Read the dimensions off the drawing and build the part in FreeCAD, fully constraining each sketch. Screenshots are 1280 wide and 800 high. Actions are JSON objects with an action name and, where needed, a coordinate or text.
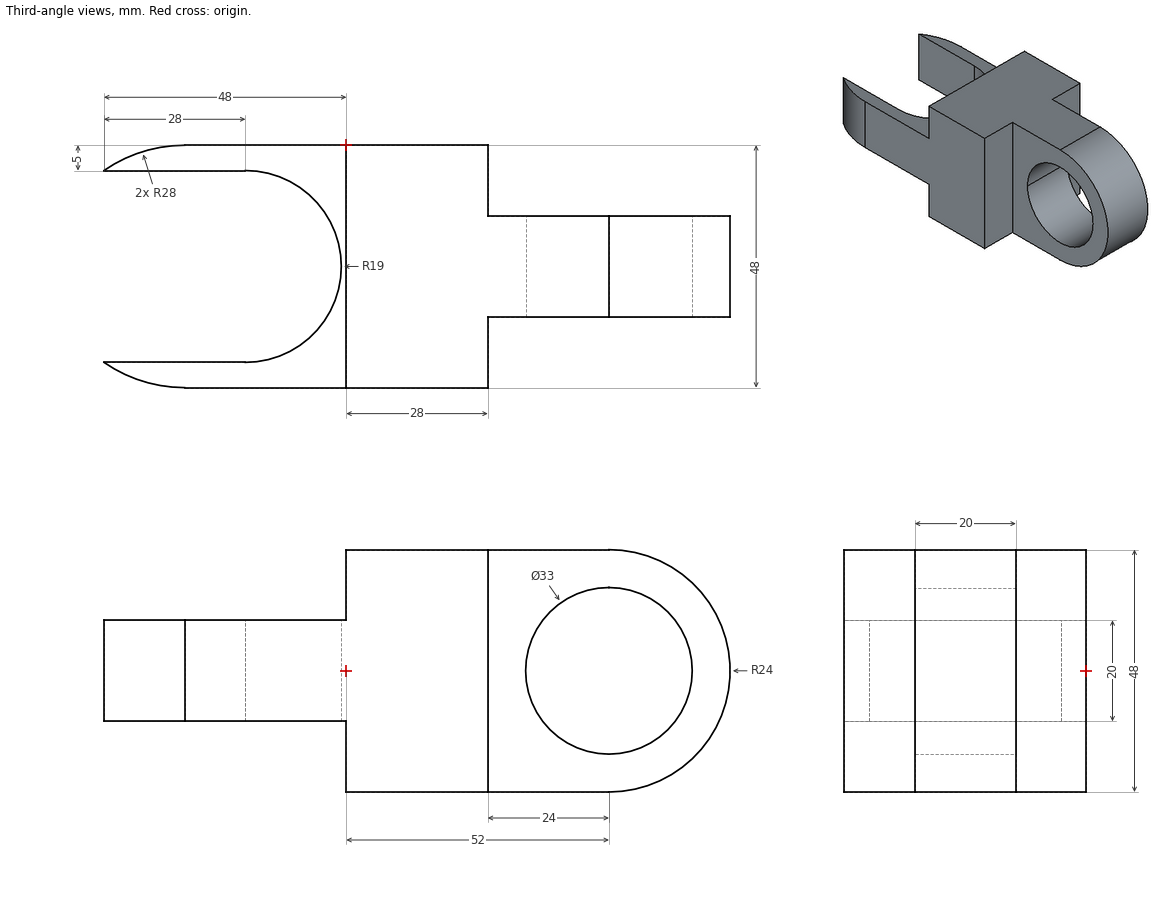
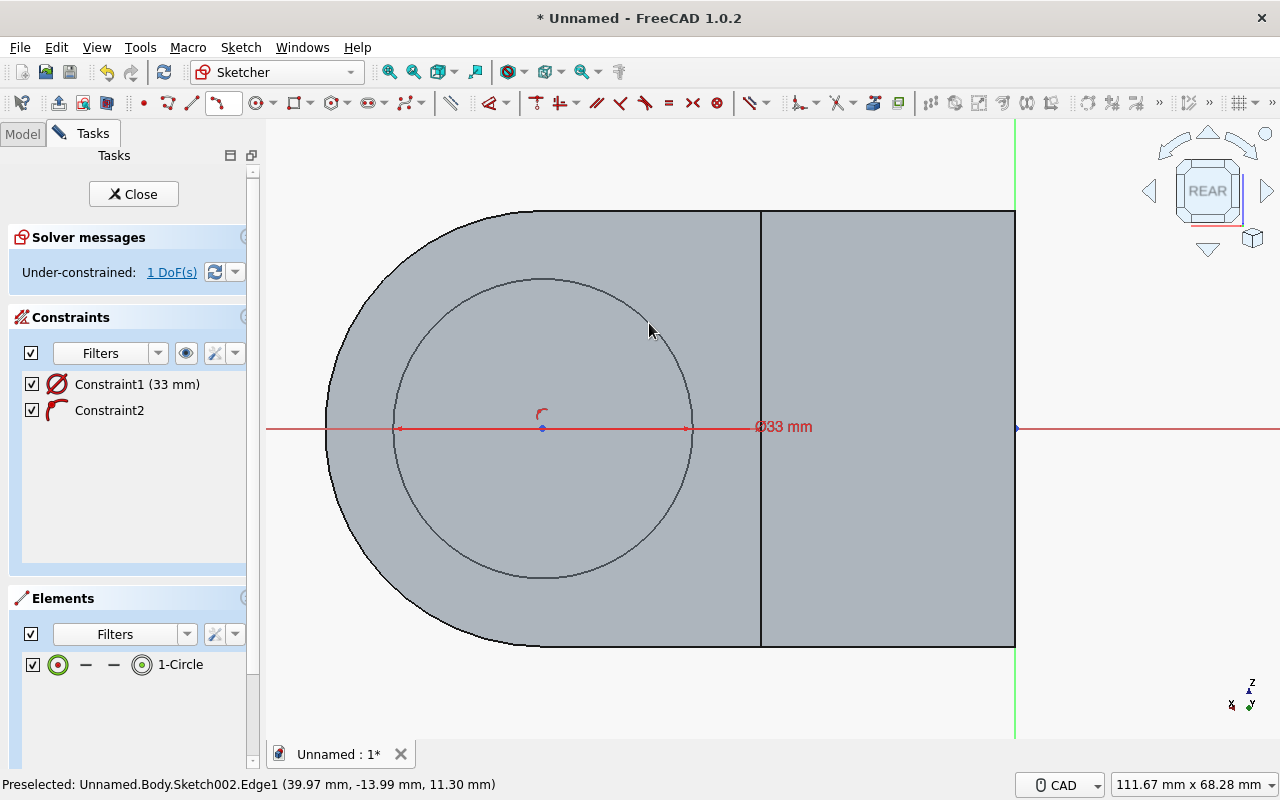
{"action": "left_click", "coordinate": [490, 104]}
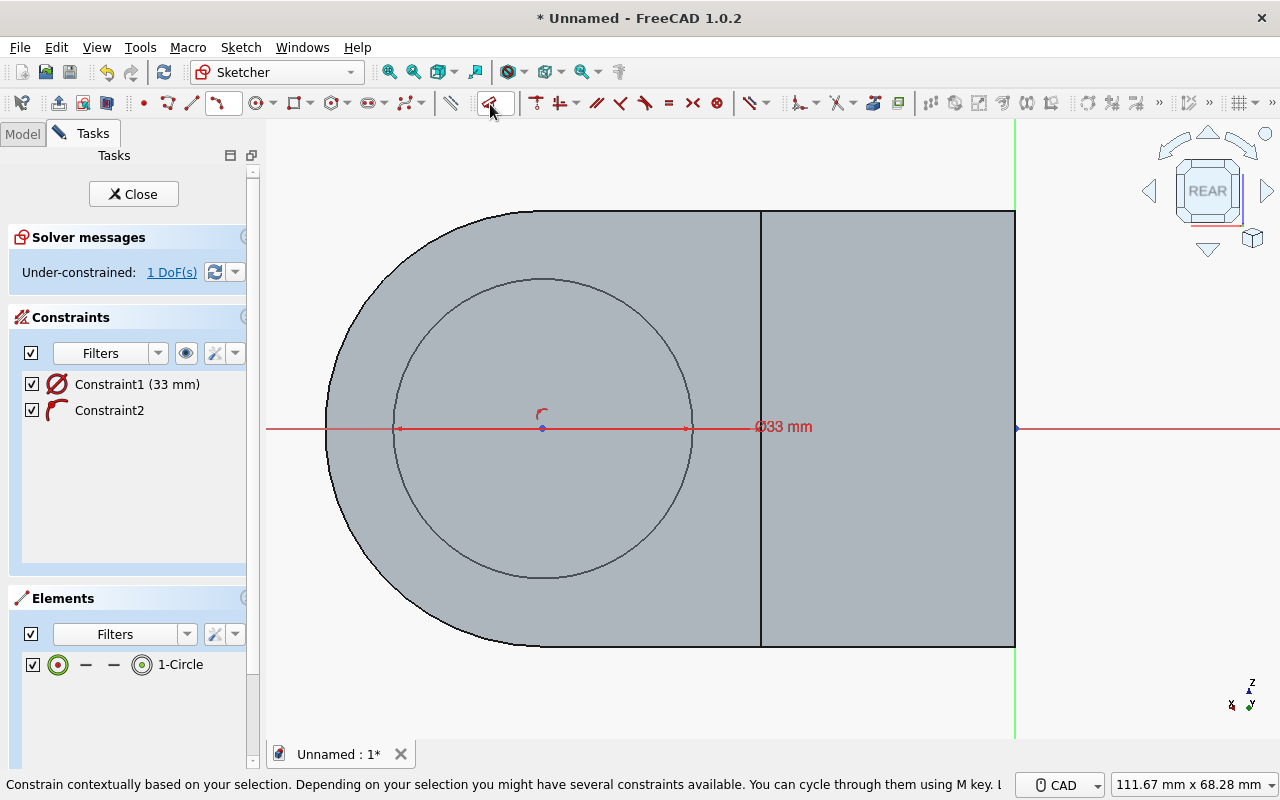
{"action": "left_click", "coordinate": [543, 429]}
{"action": "left_click", "coordinate": [779, 463]}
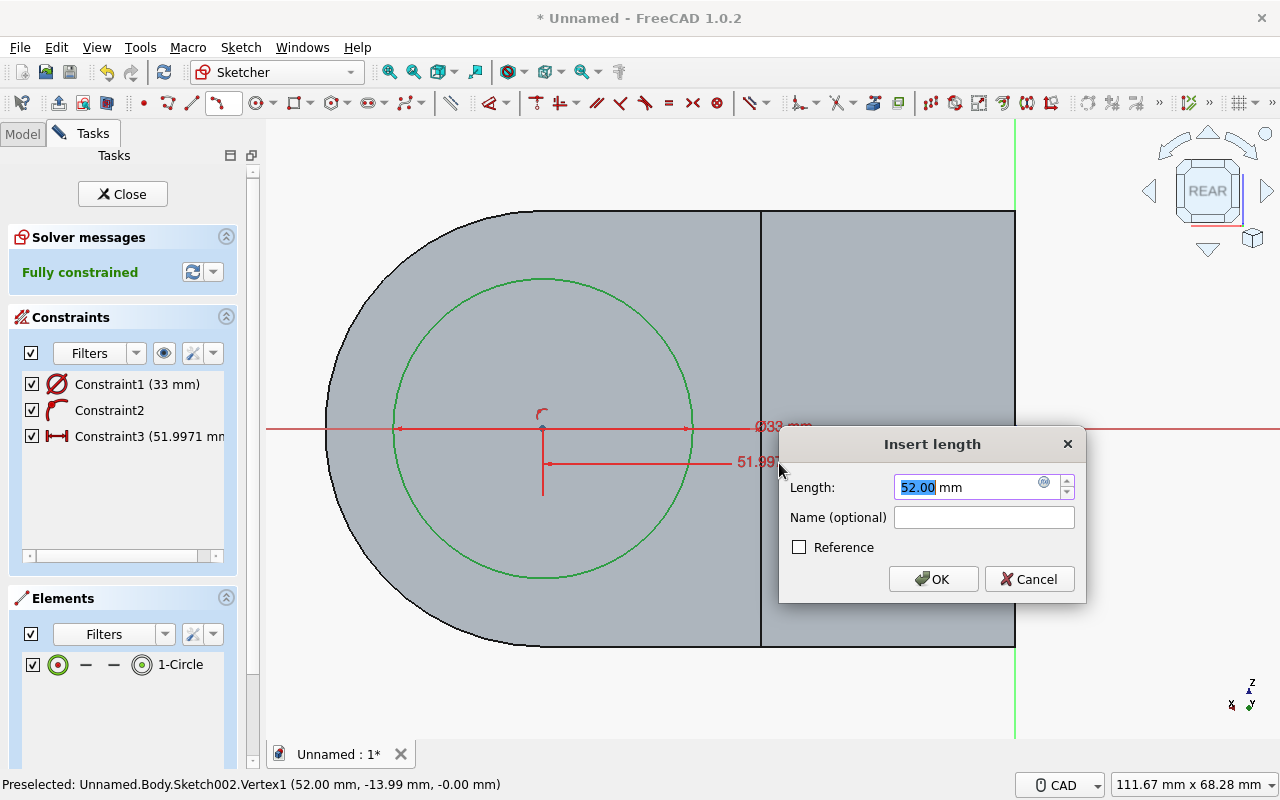
{"action": "type", "text": "52"}
{"action": "key", "text": "Return"}
{"action": "key", "text": "Escape"}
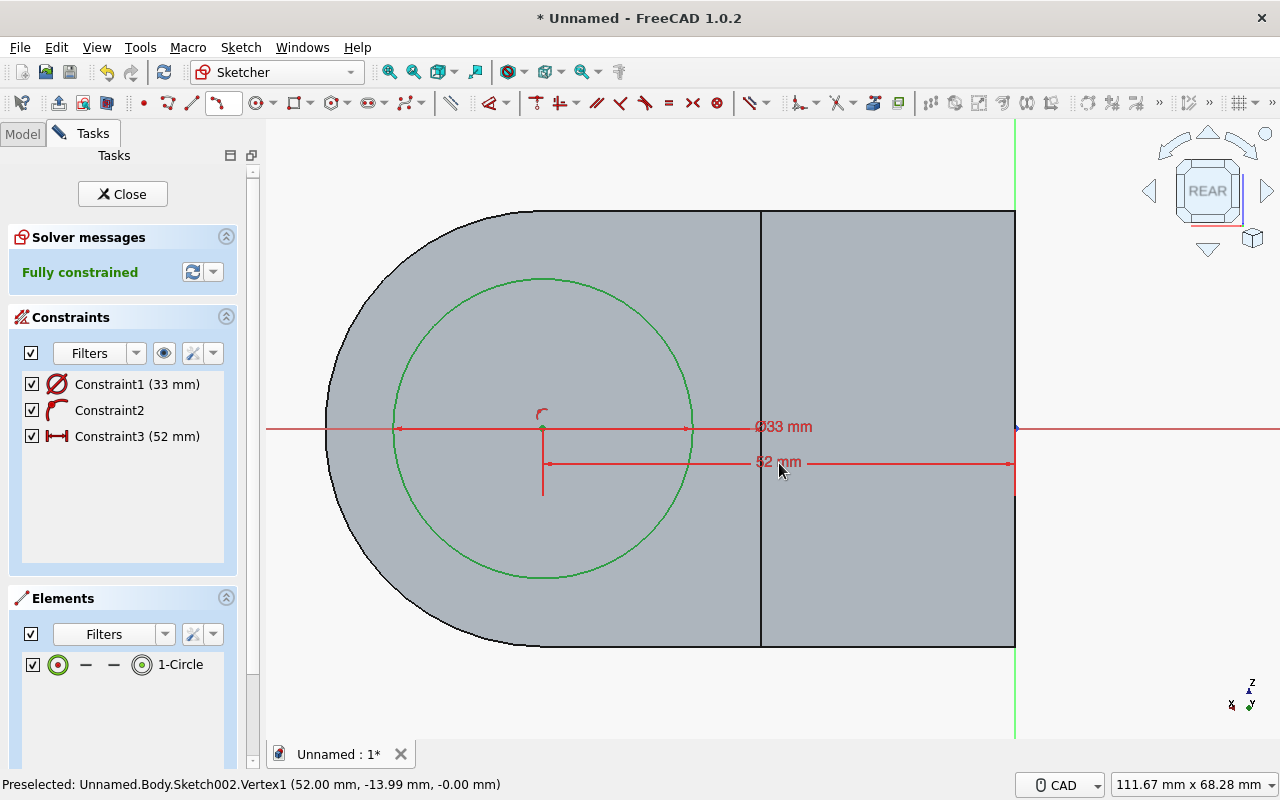
{"action": "left_click", "coordinate": [123, 194]}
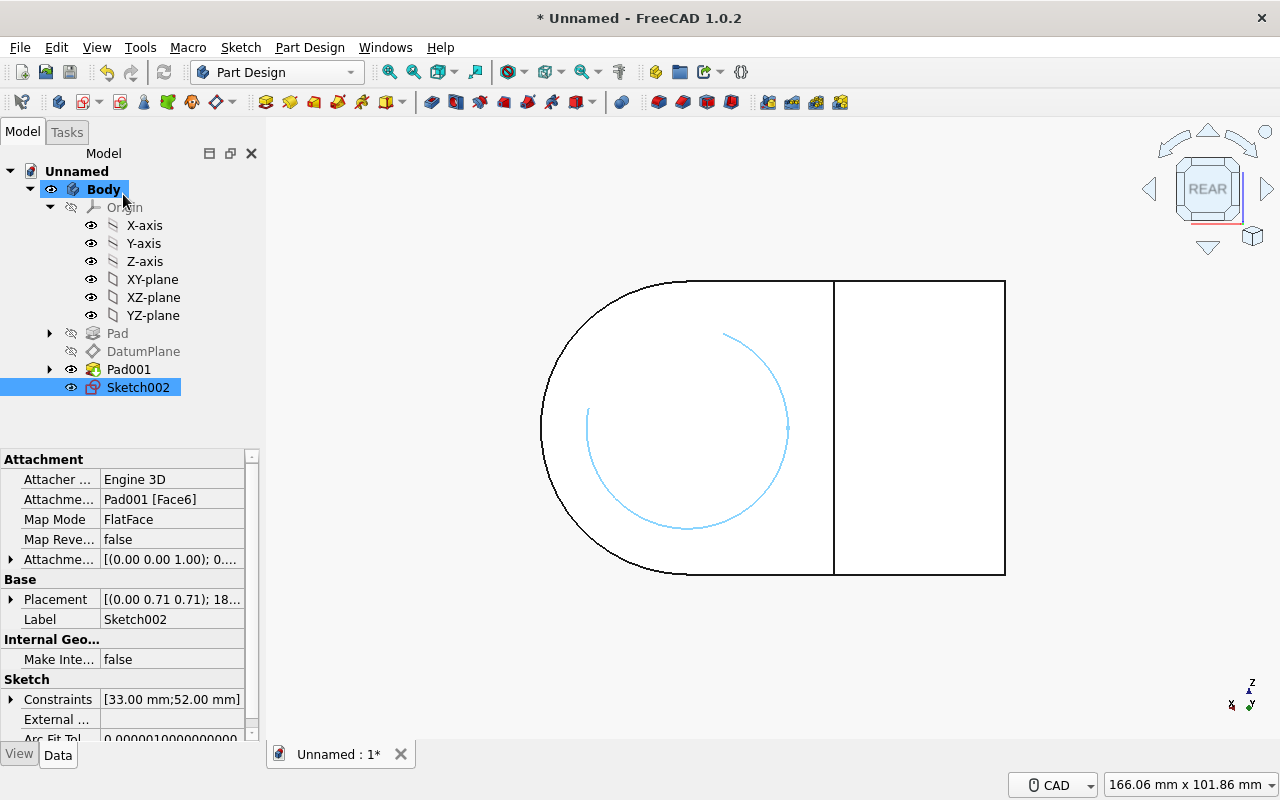
{"action": "left_click", "coordinate": [432, 102]}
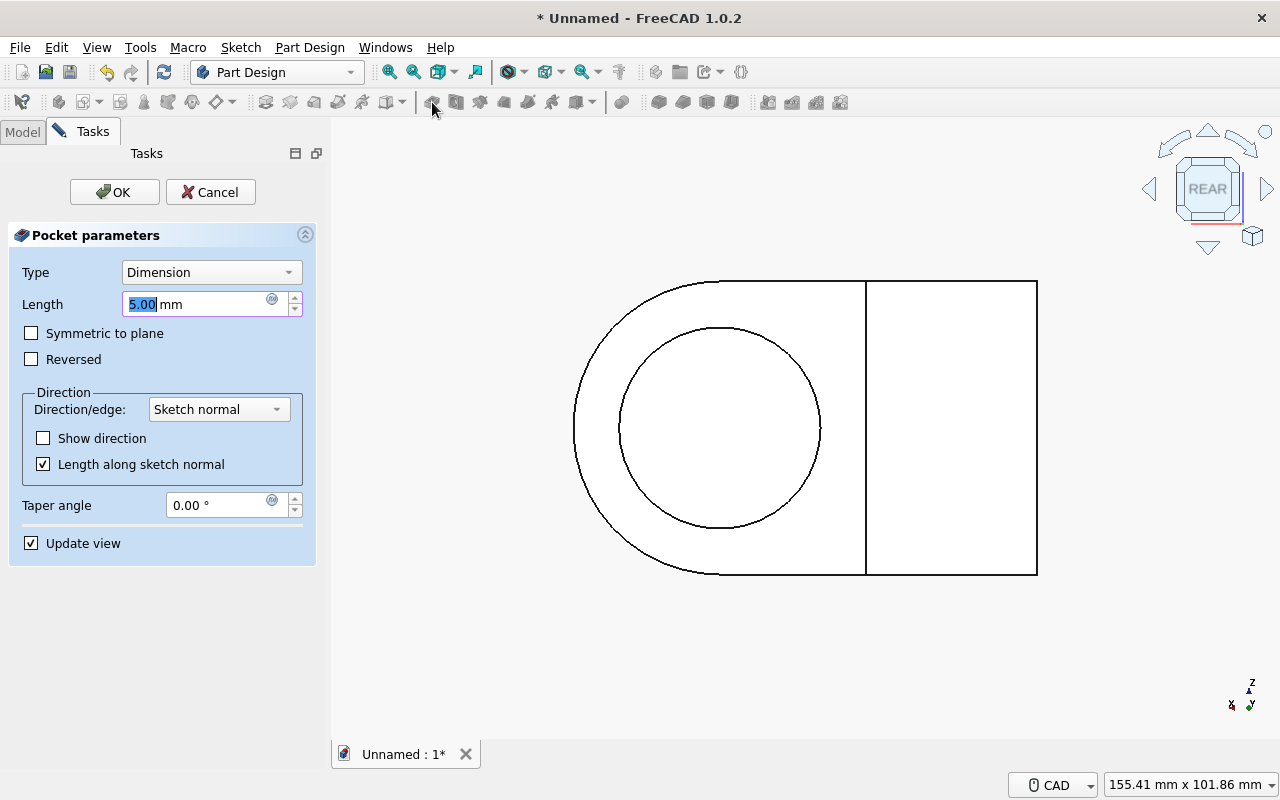
{"action": "type", "text": "20"}
{"action": "key", "text": "Tab"}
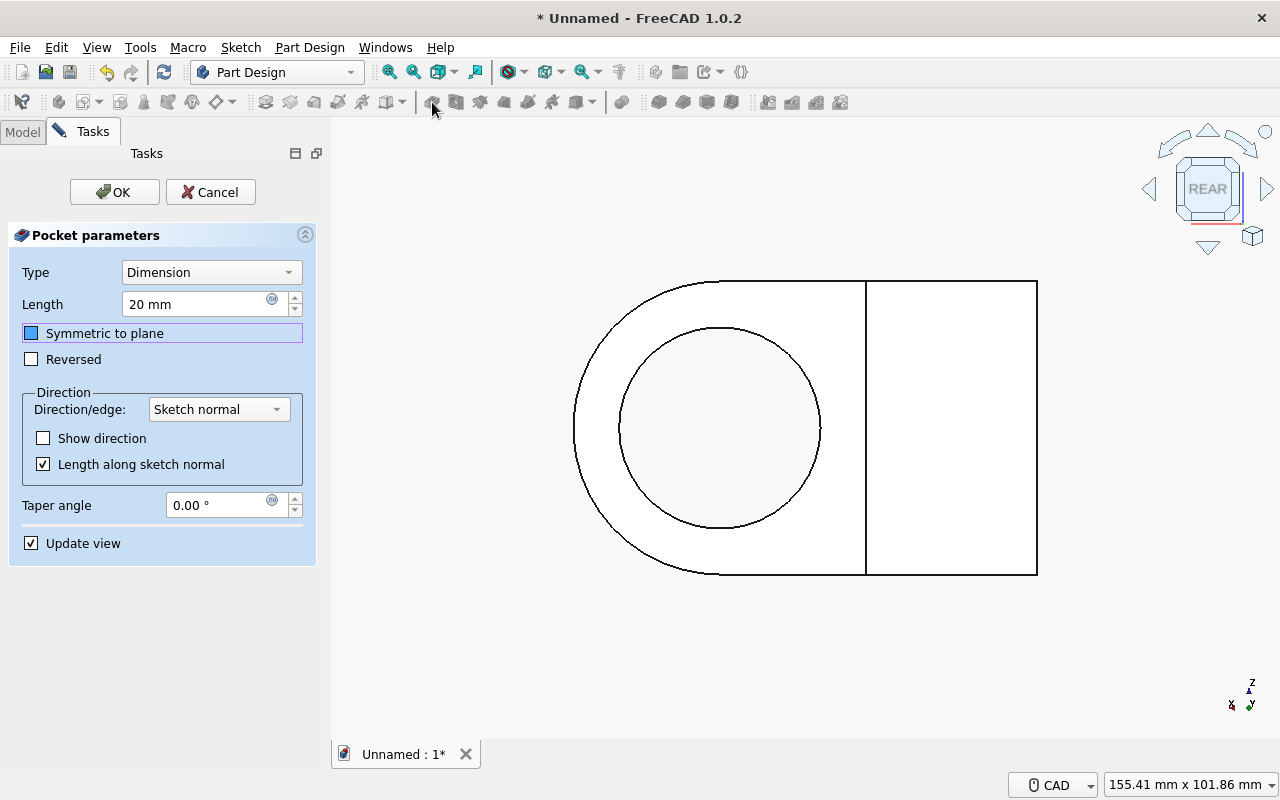
{"action": "left_click", "coordinate": [115, 192]}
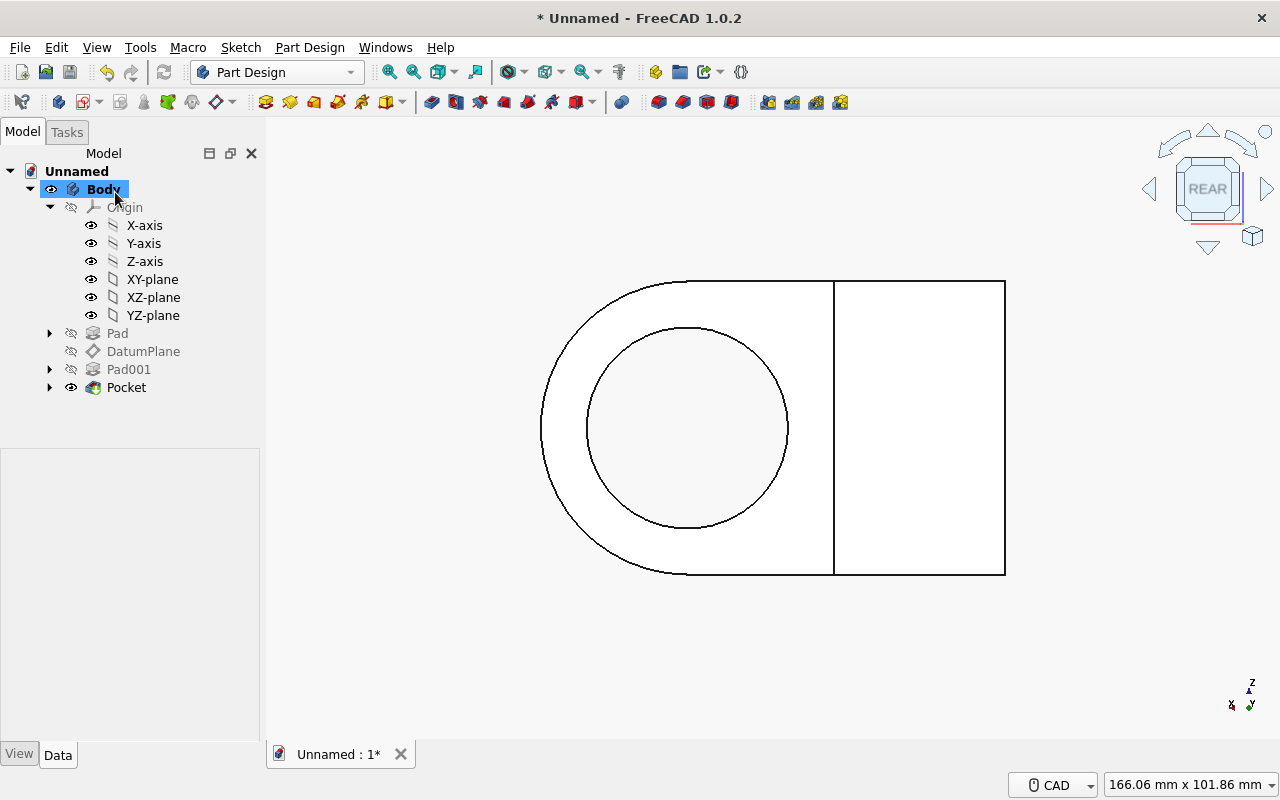
{"action": "left_click", "coordinate": [84, 102]}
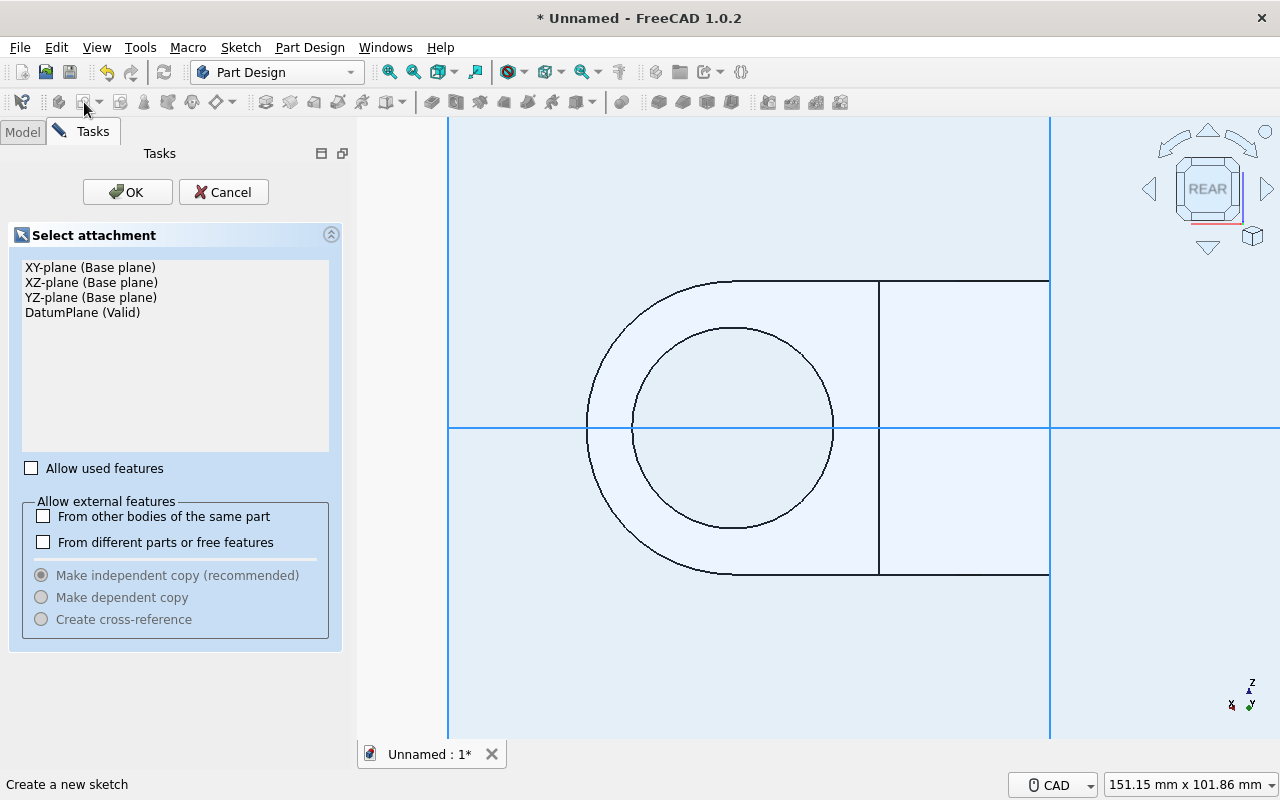
{"action": "left_click", "coordinate": [82, 268]}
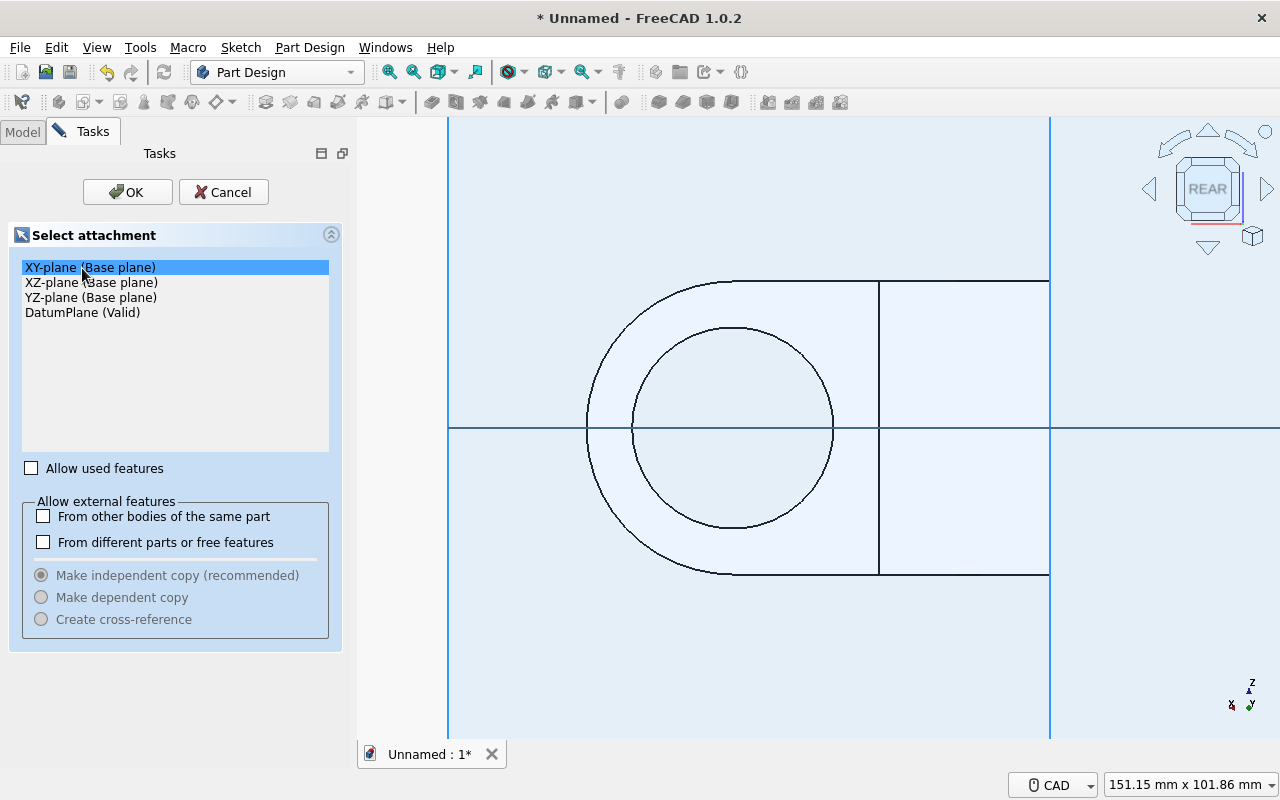
{"action": "left_click", "coordinate": [128, 192]}